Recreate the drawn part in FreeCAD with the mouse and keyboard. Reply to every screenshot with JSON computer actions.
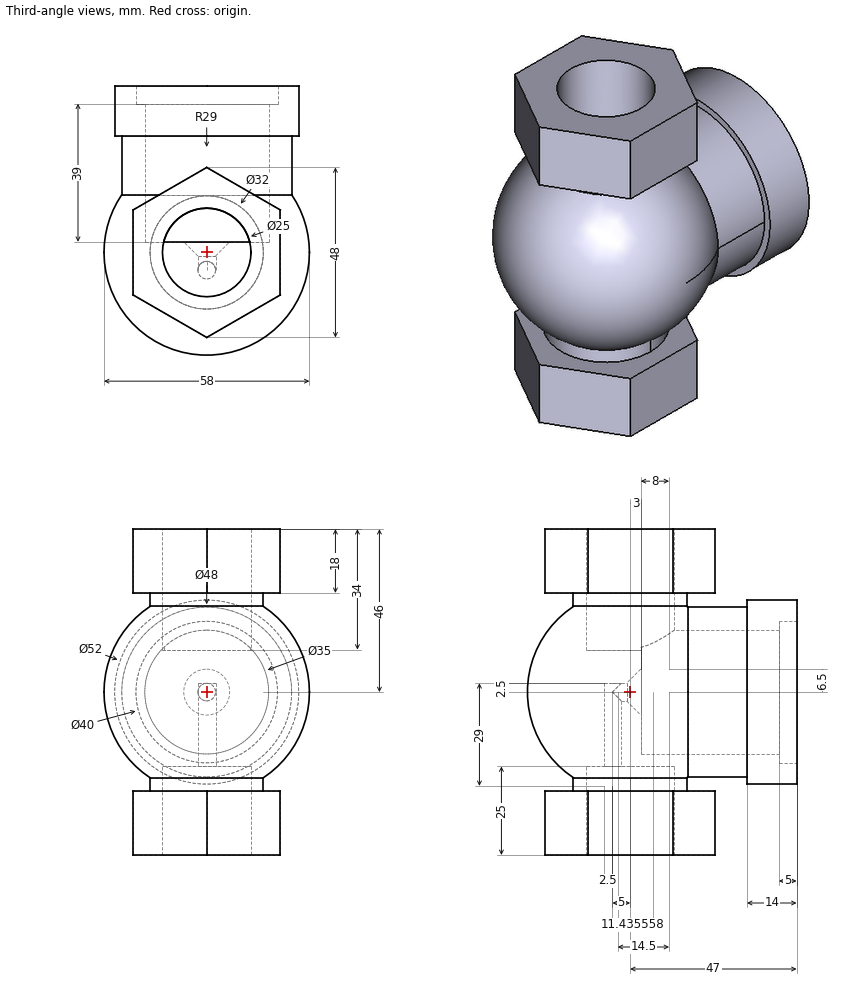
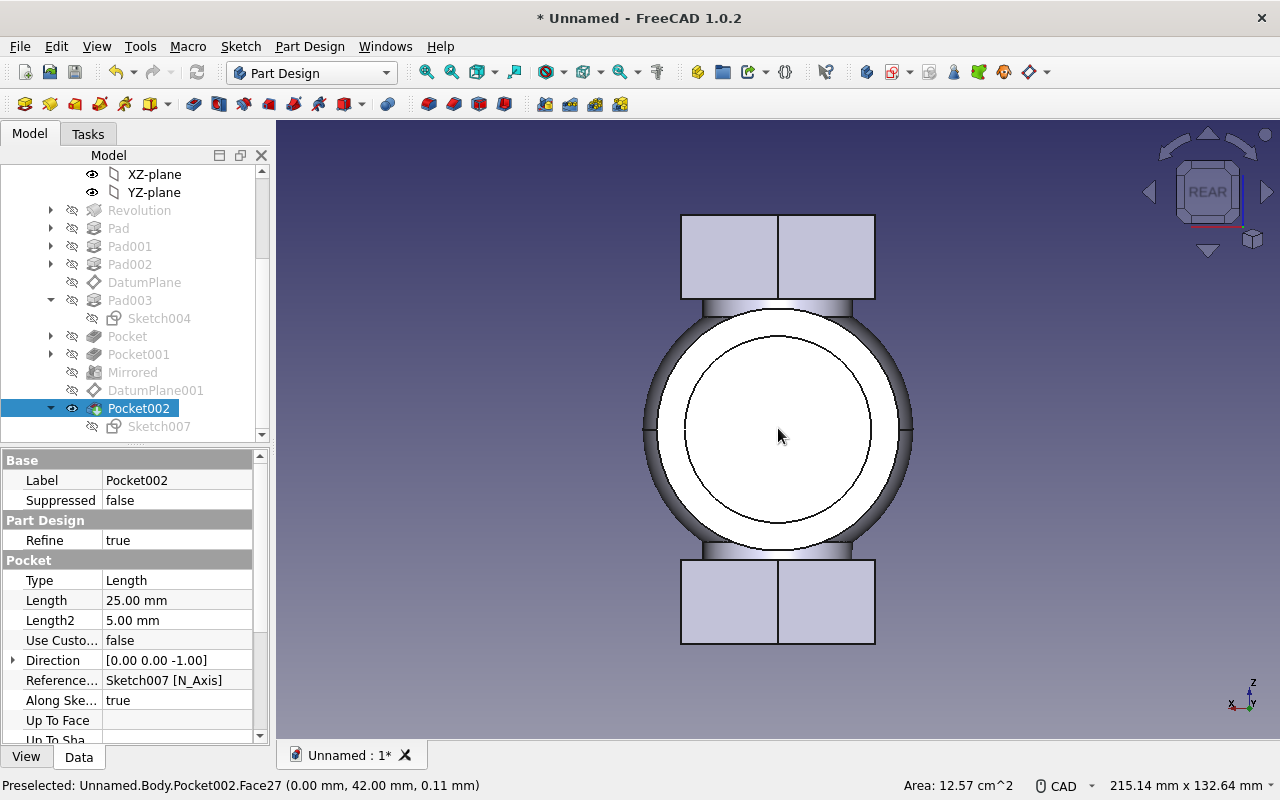
{"action": "left_click", "coordinate": [892, 72]}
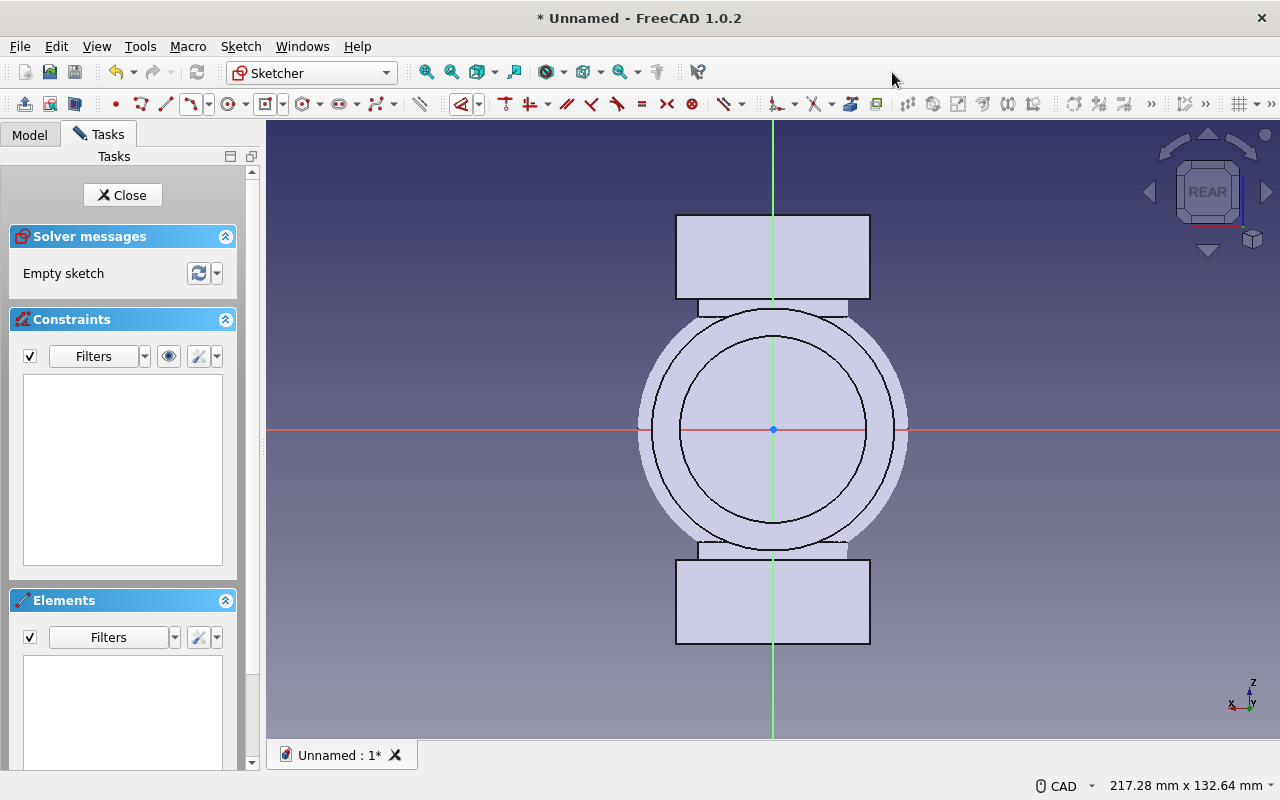
{"action": "scroll", "coordinate": [829, 429], "scroll_direction": "up", "scroll_amount": 4}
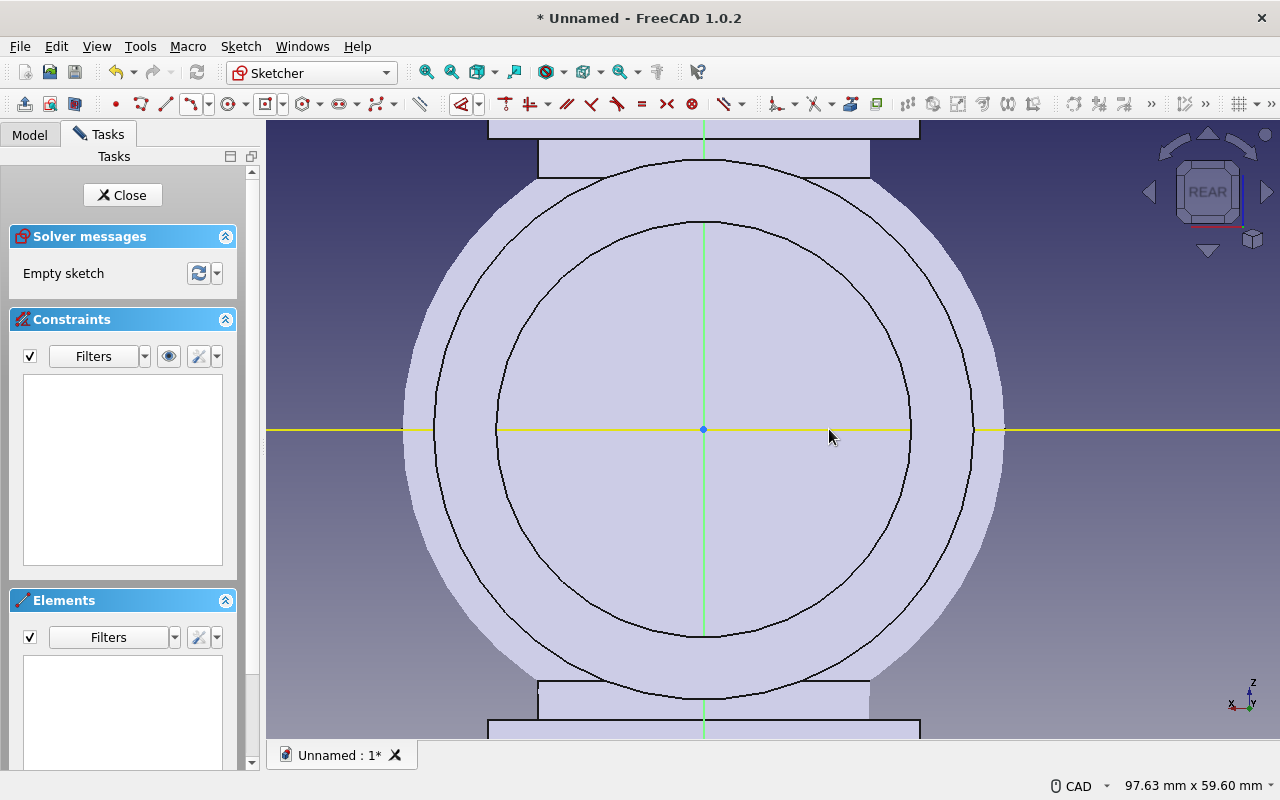
{"action": "key", "text": "g c"}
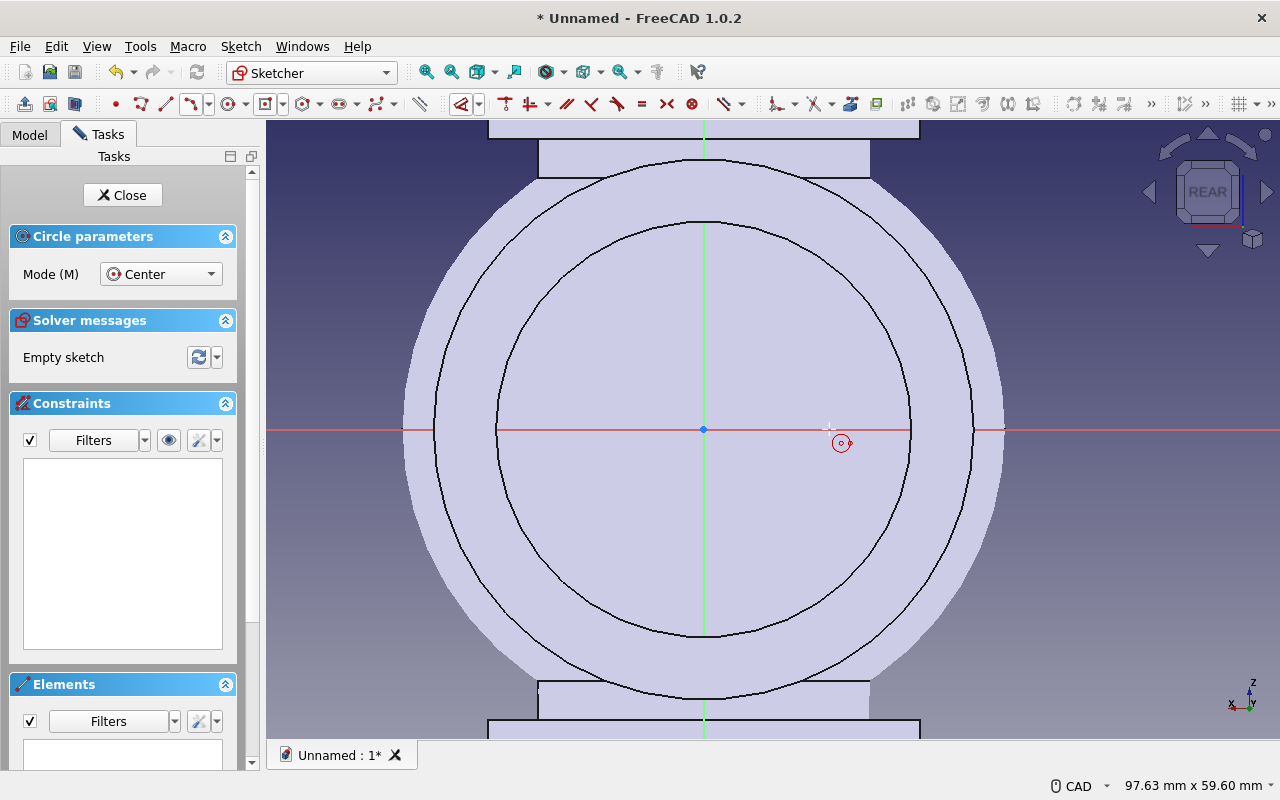
{"action": "left_click", "coordinate": [704, 429]}
{"action": "left_click", "coordinate": [832, 301]}
{"action": "key", "text": "Escape"}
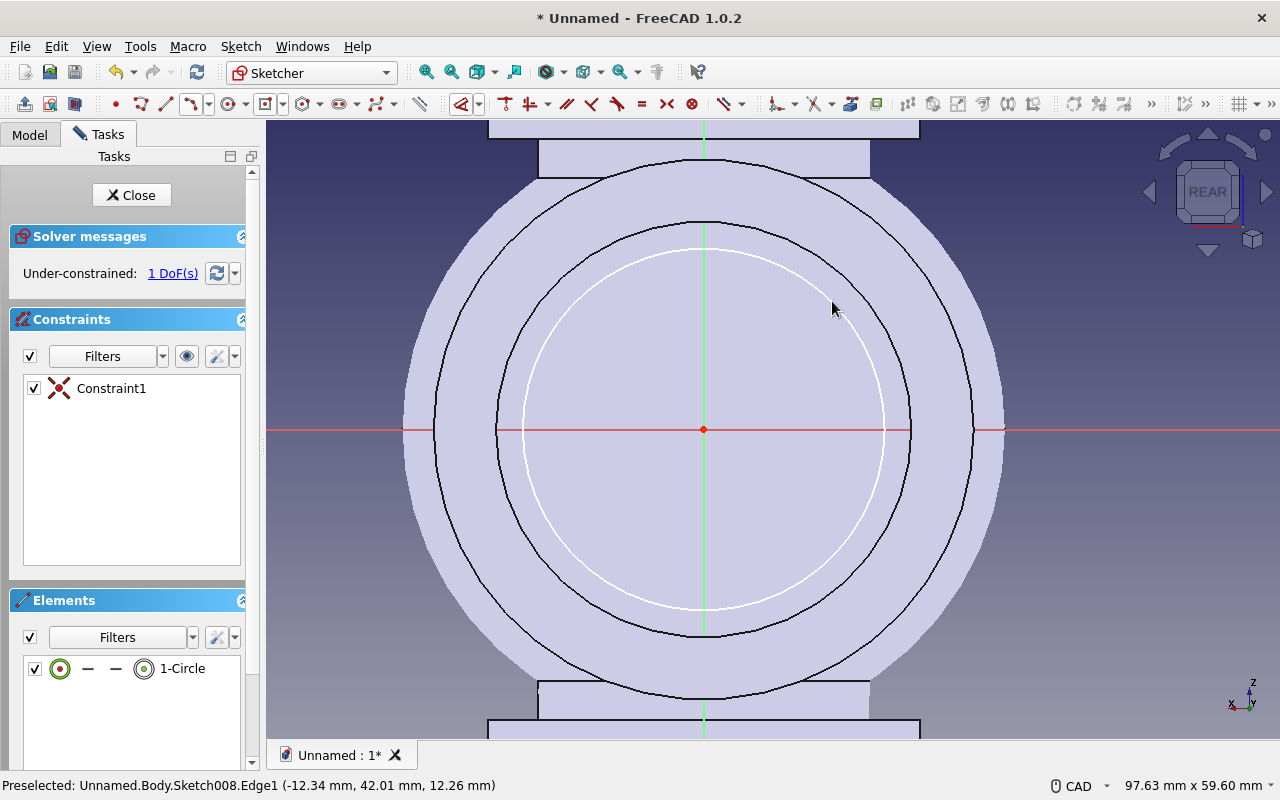
{"action": "left_click", "coordinate": [831, 301]}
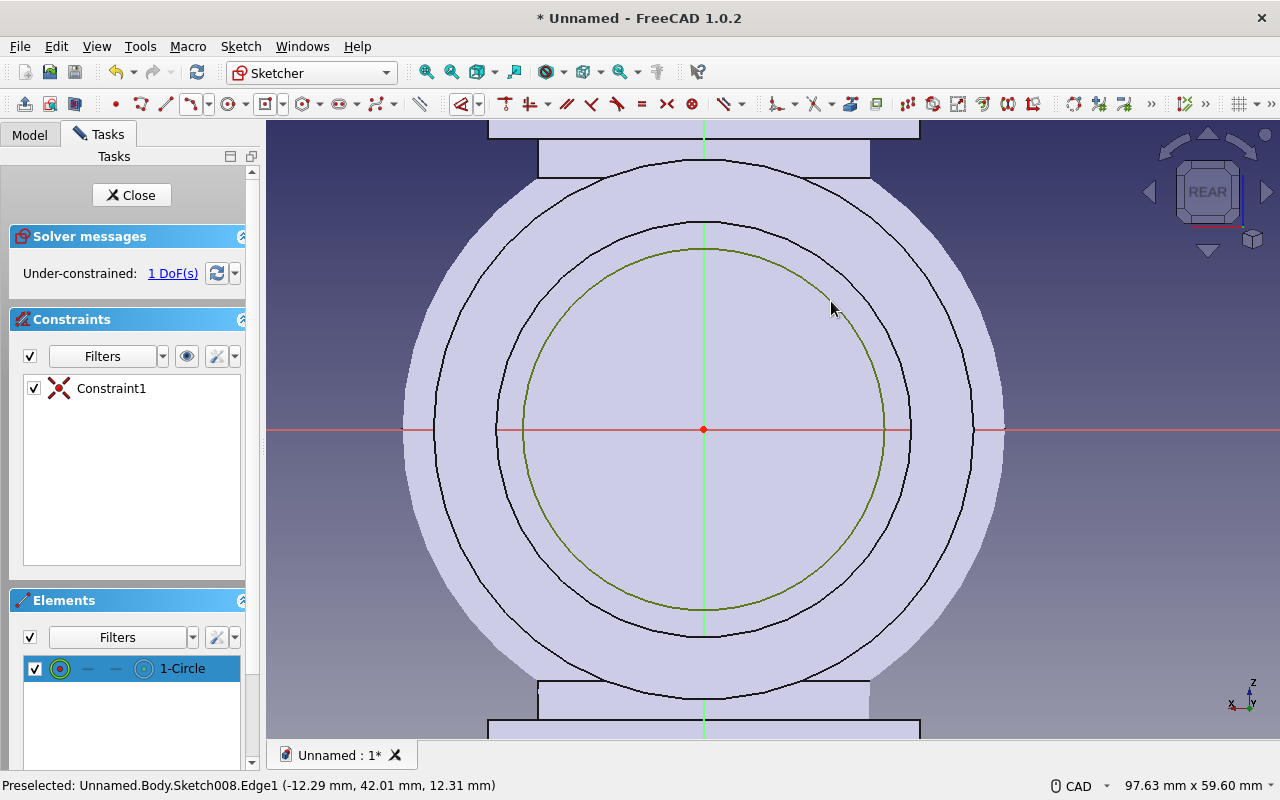
{"action": "left_click", "coordinate": [478, 104]}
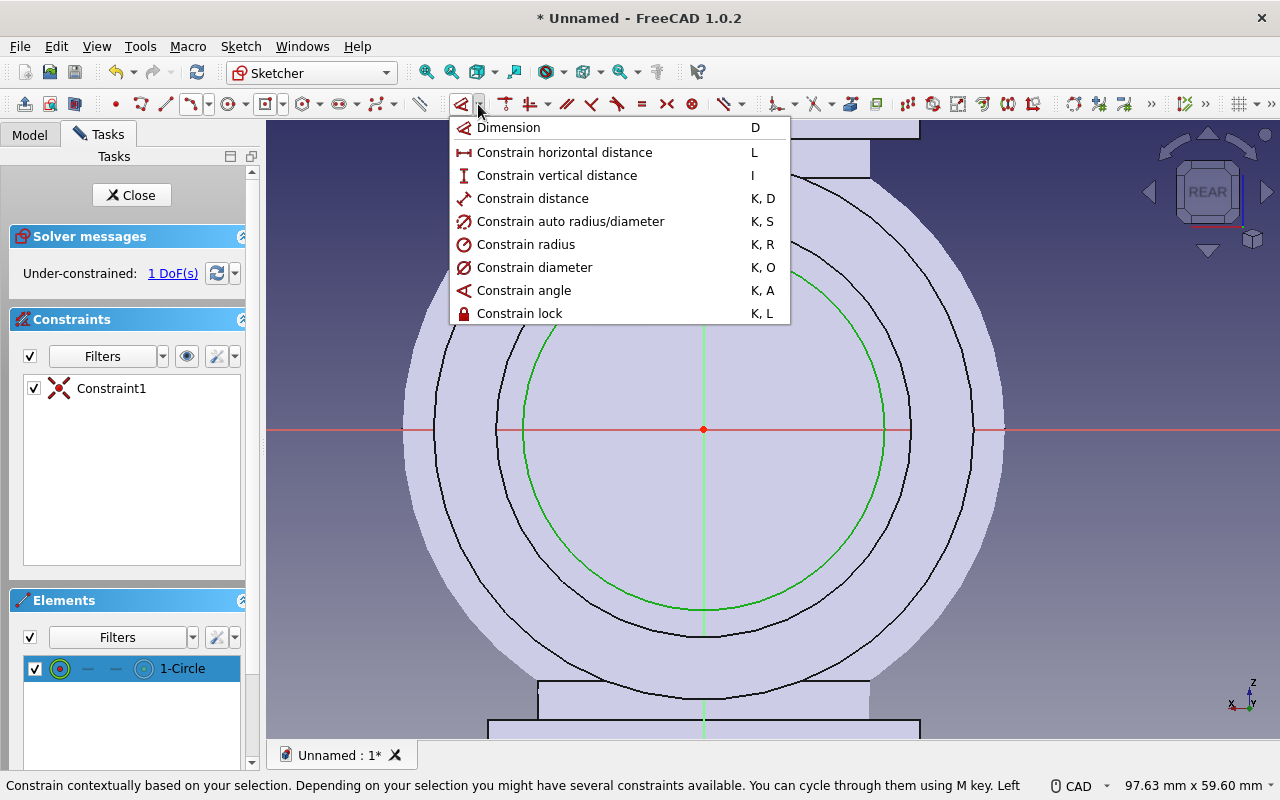
{"action": "left_click", "coordinate": [620, 268]}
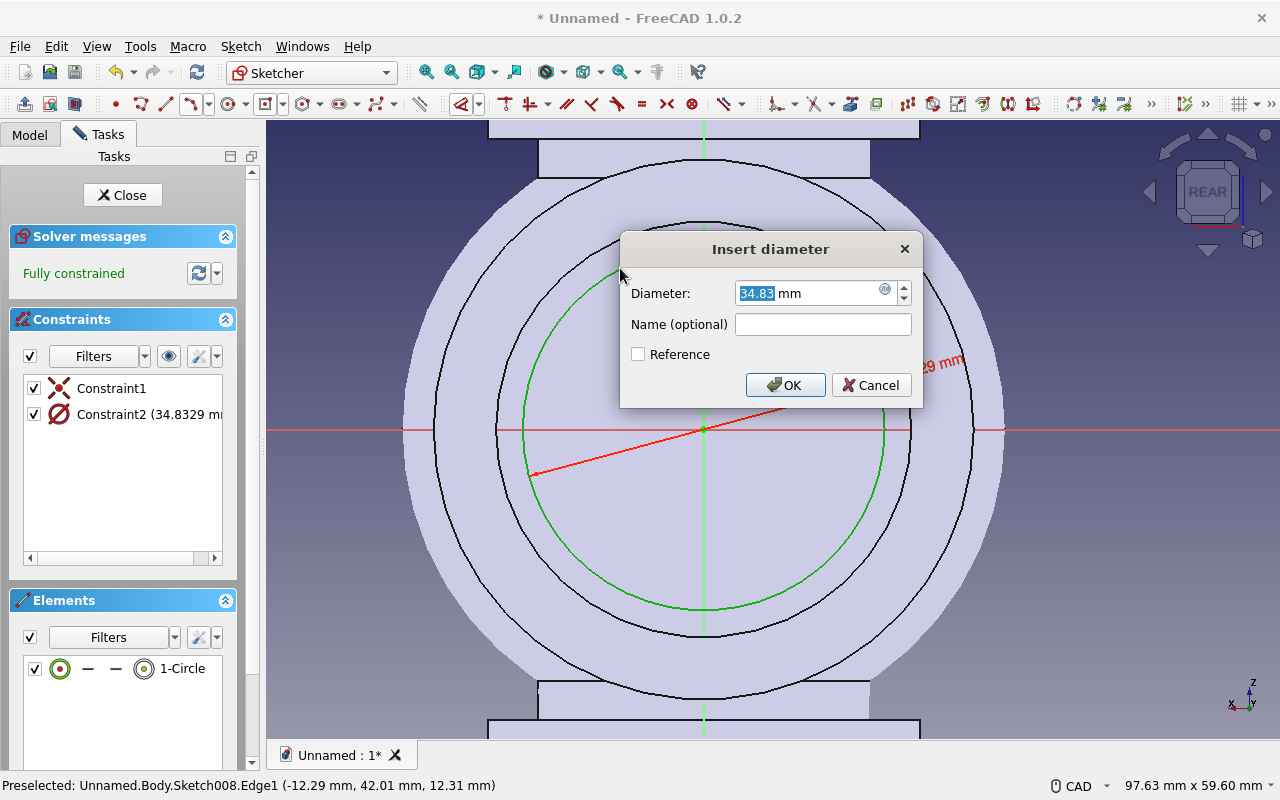
{"action": "type", "text": "35"}
{"action": "key", "text": "Return"}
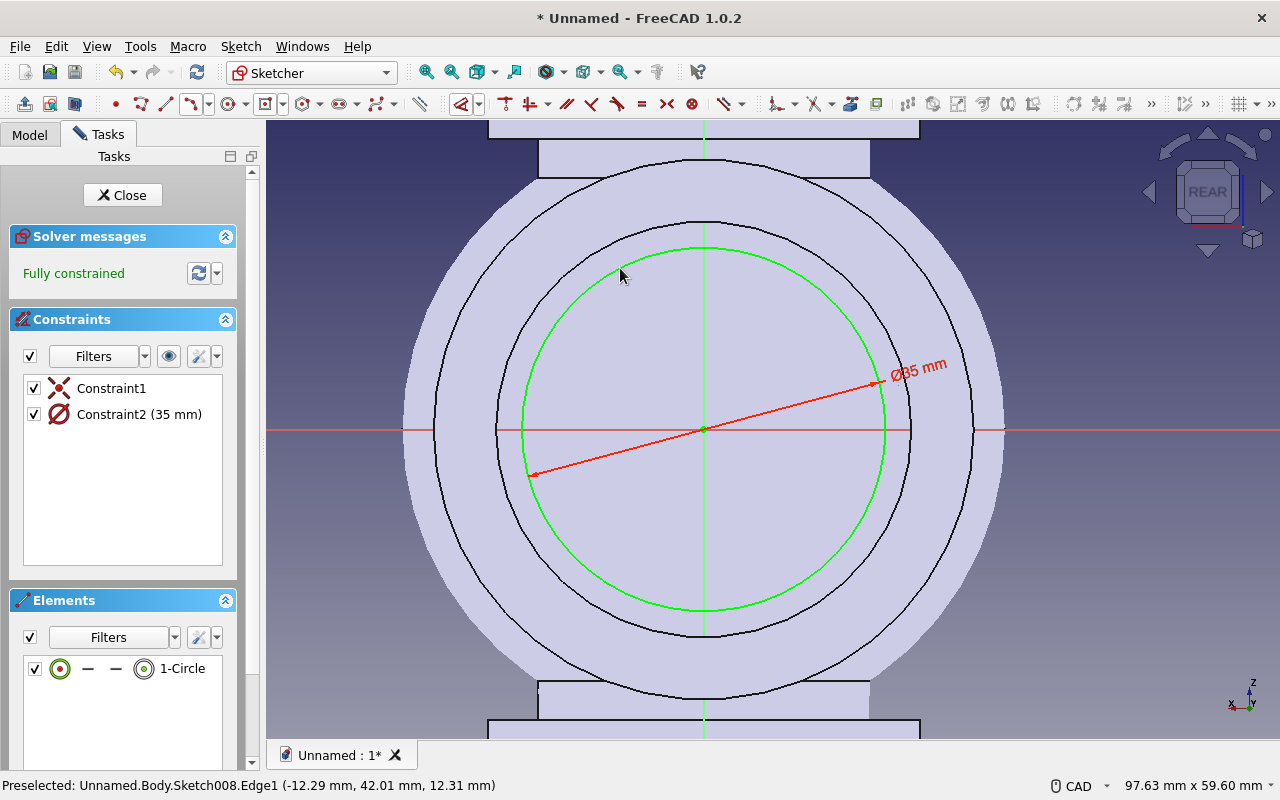
{"action": "left_click", "coordinate": [123, 195]}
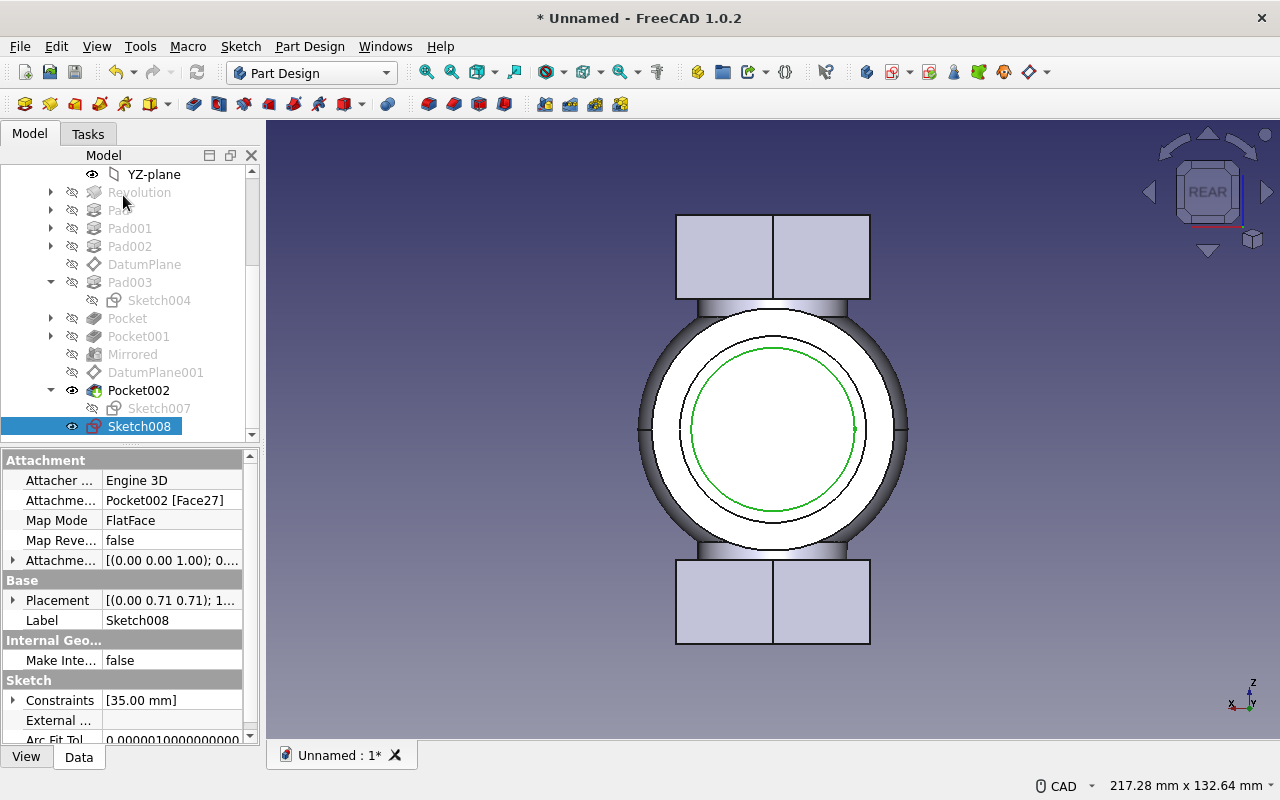
{"action": "left_click", "coordinate": [194, 104]}